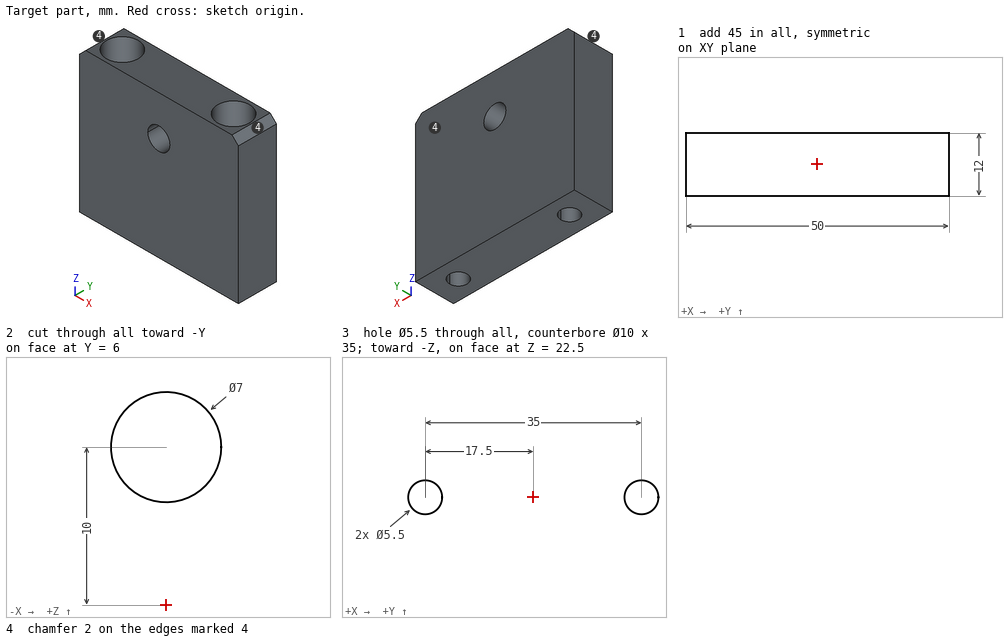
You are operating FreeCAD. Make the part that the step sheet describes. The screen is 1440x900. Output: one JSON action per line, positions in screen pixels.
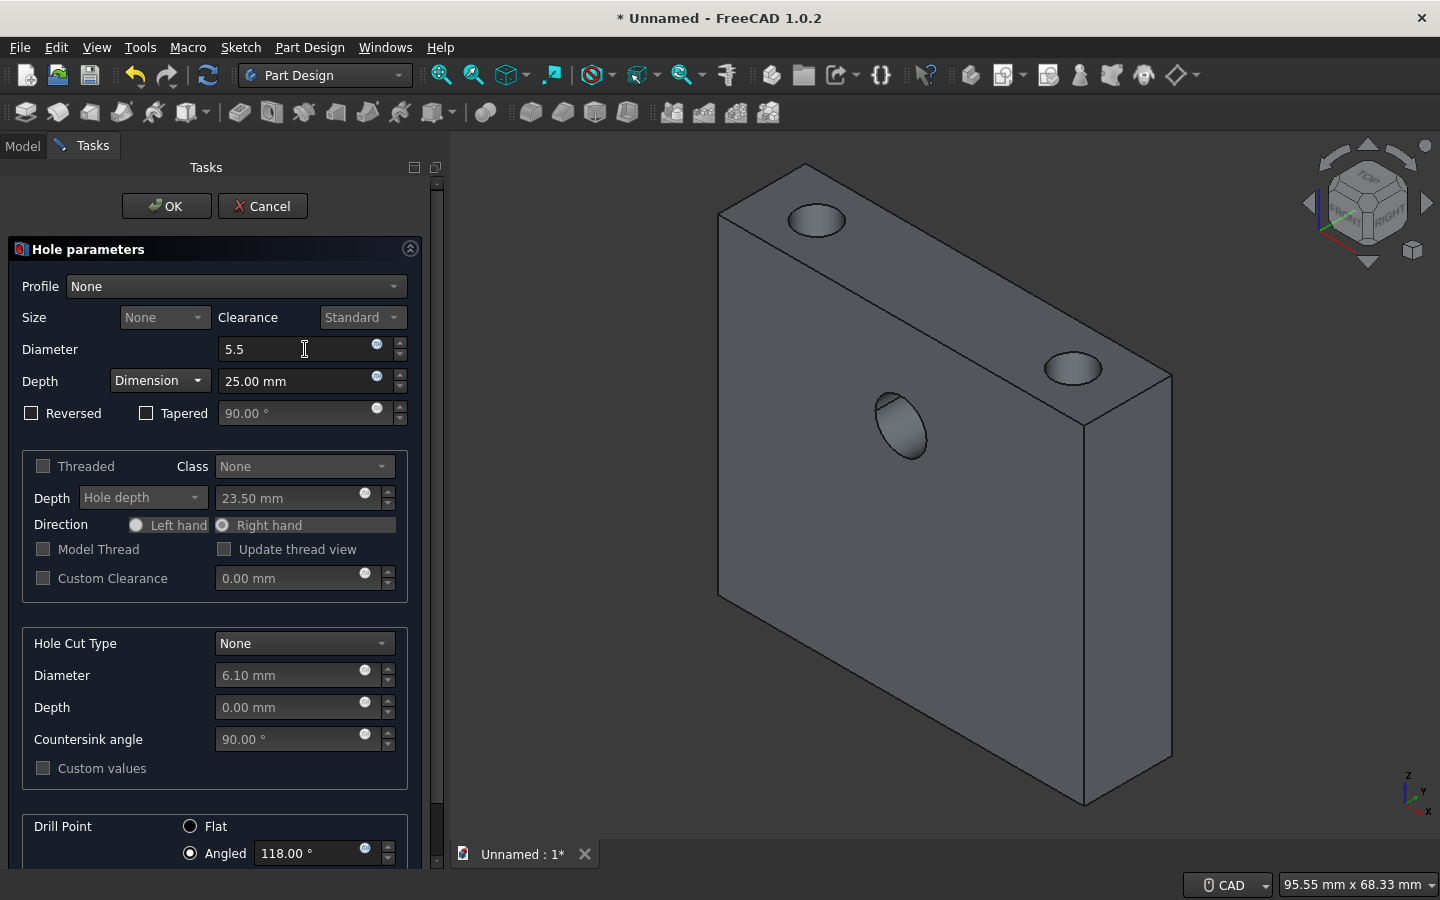
{"action": "left_click", "coordinate": [161, 380]}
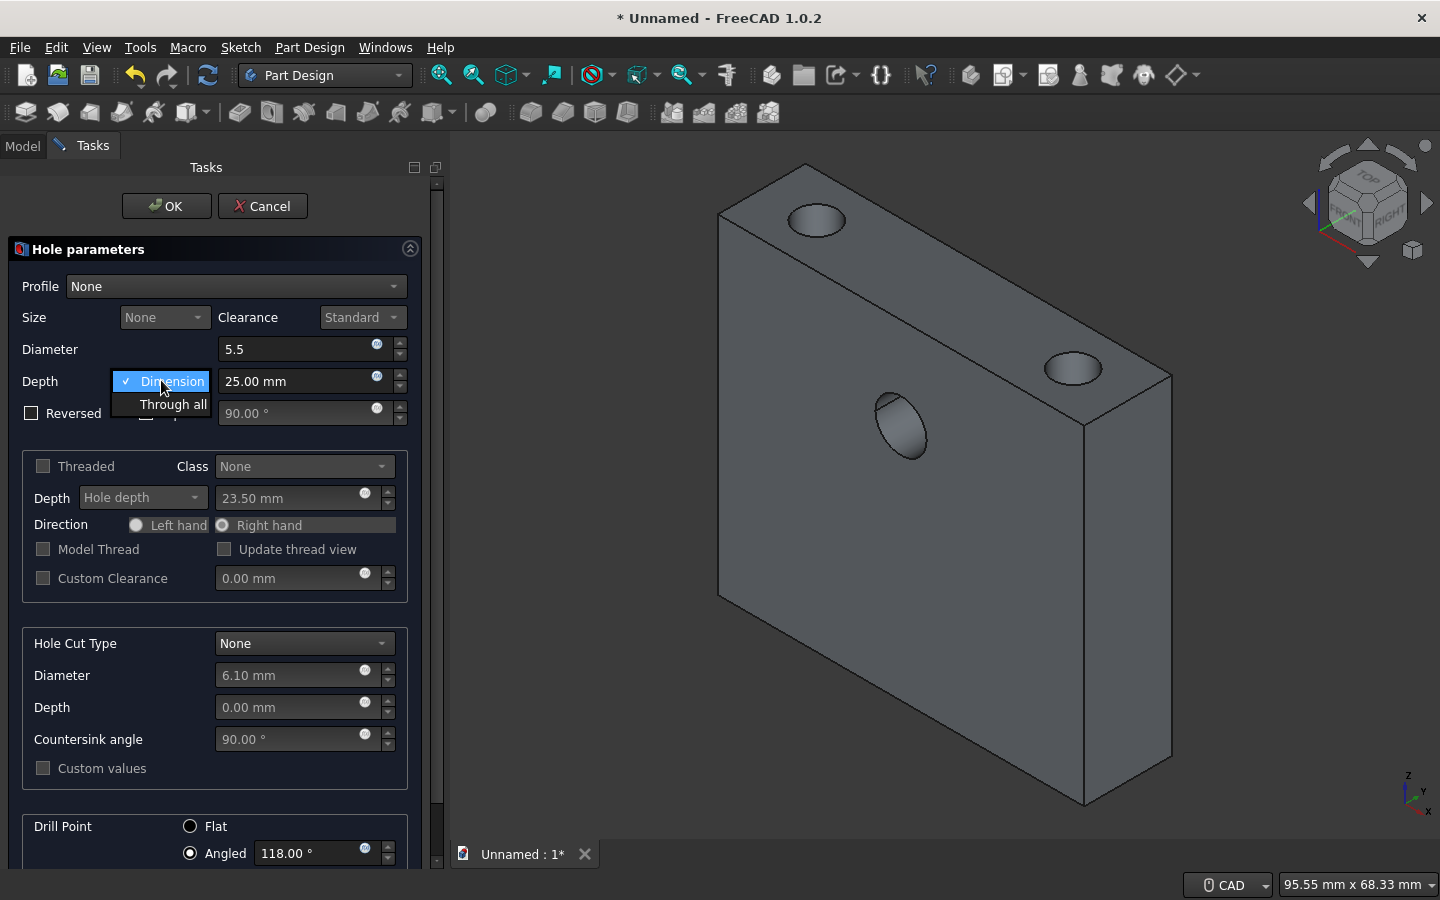
{"action": "left_click", "coordinate": [160, 404]}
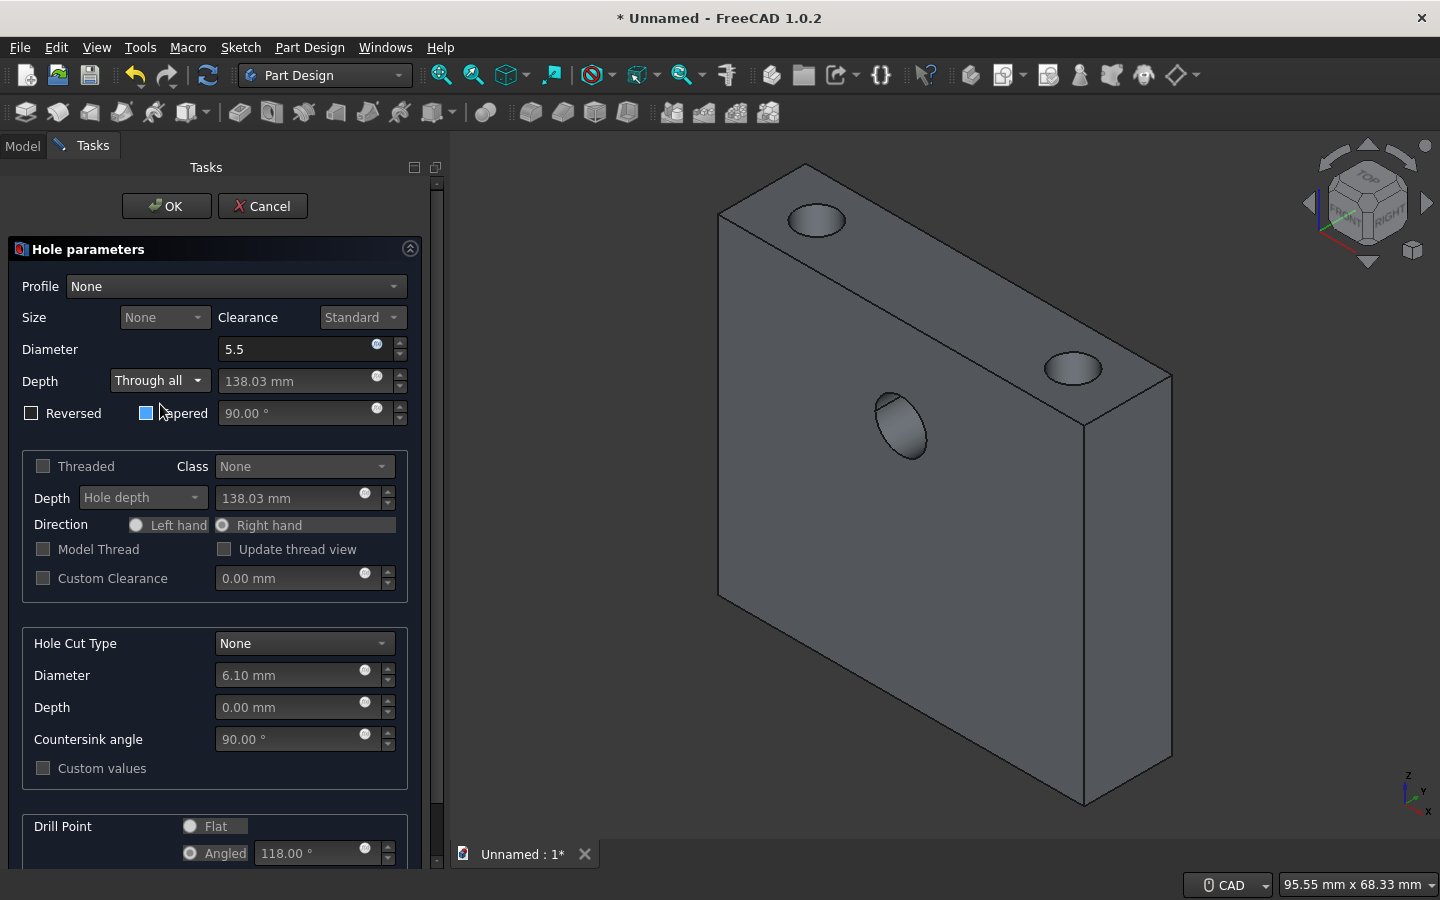
{"action": "left_click", "coordinate": [306, 644]}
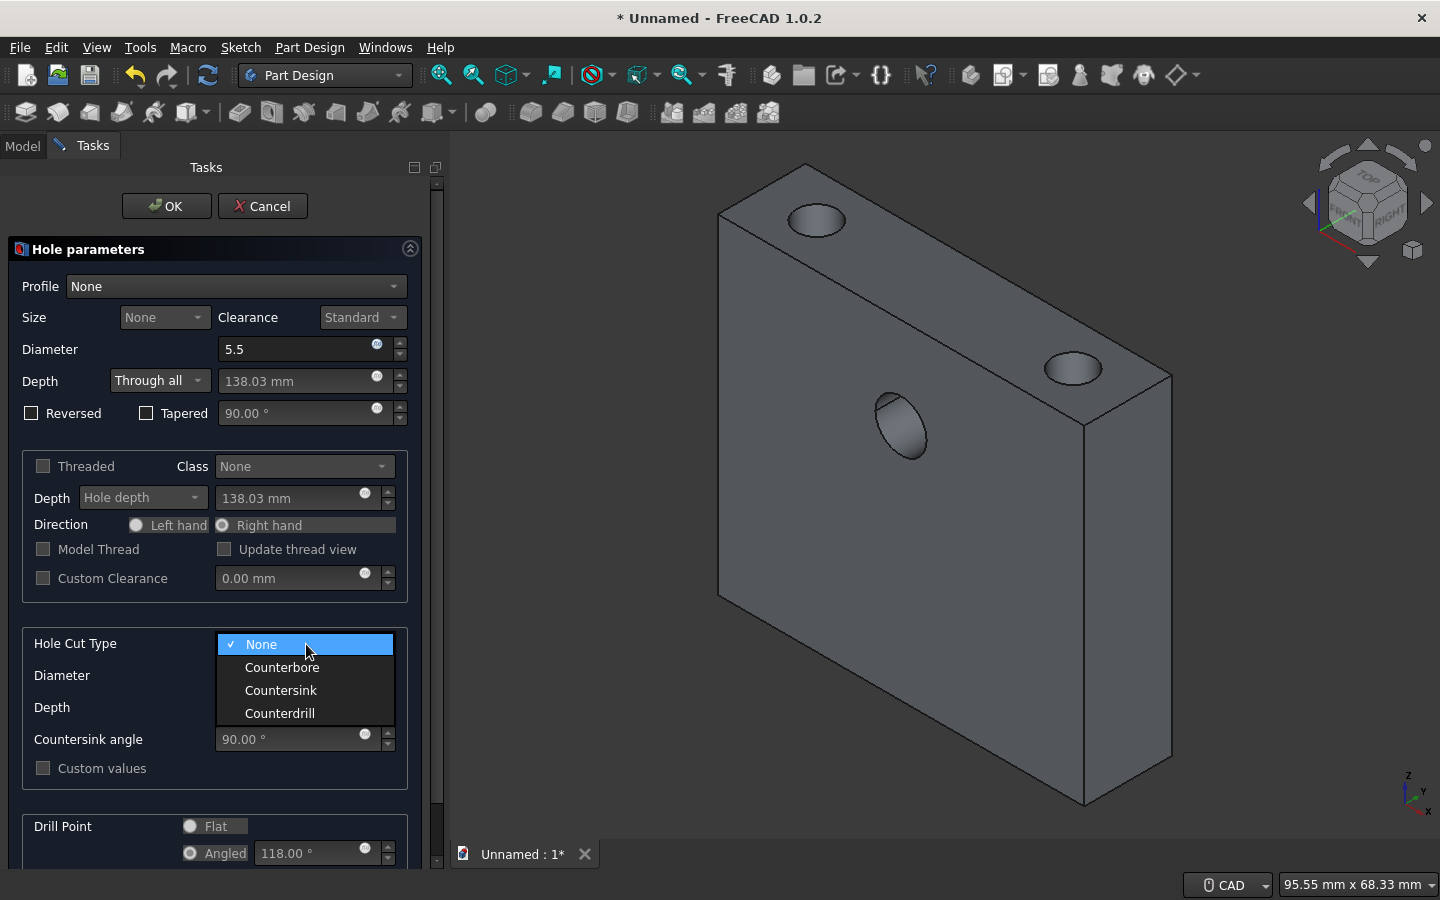
{"action": "left_click", "coordinate": [304, 668]}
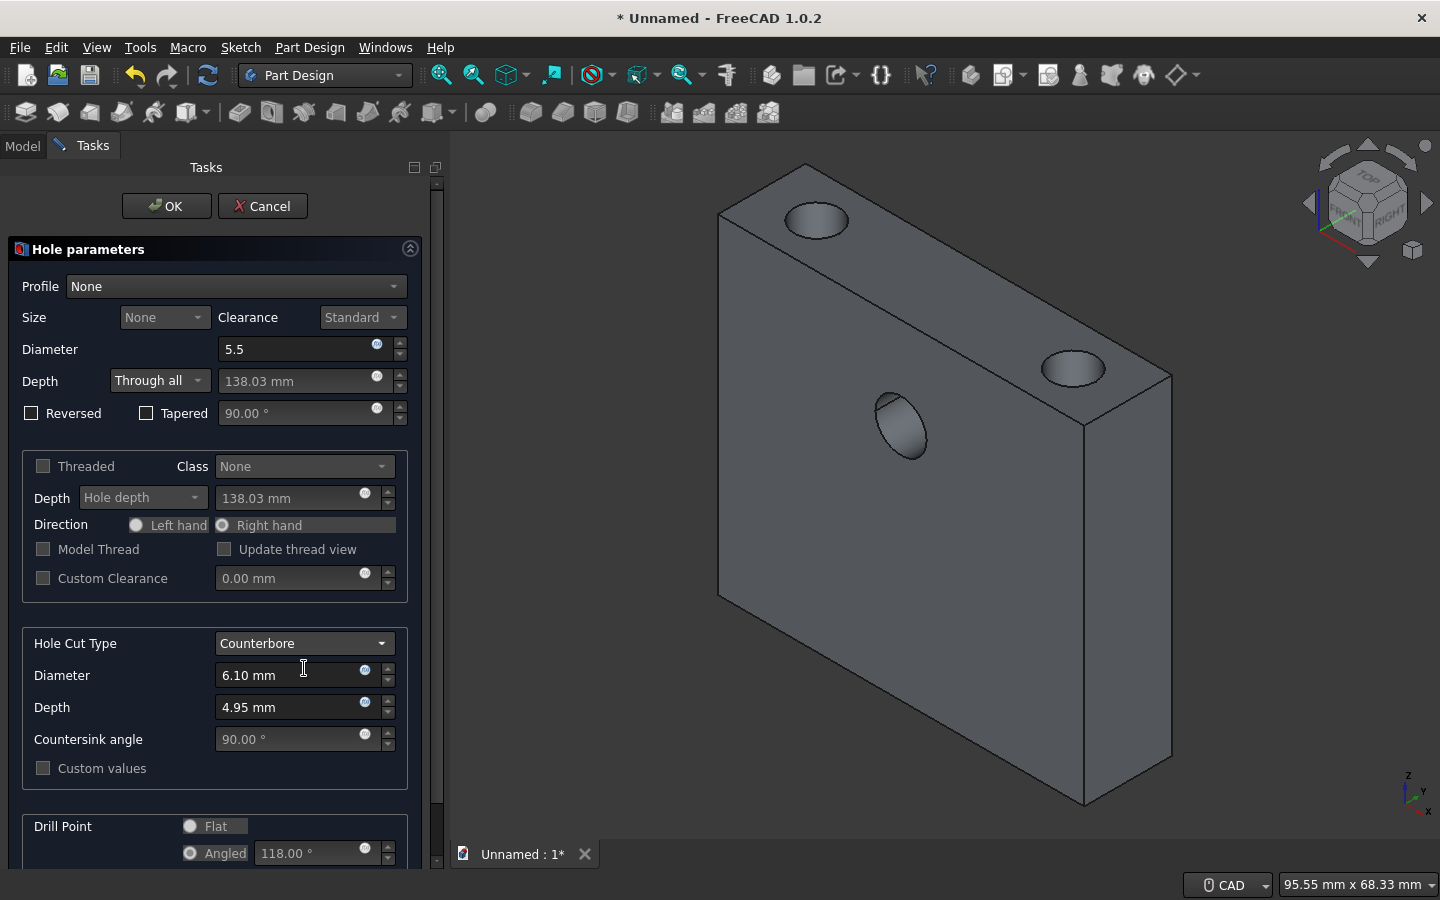
{"action": "triple_click", "coordinate": [298, 675]}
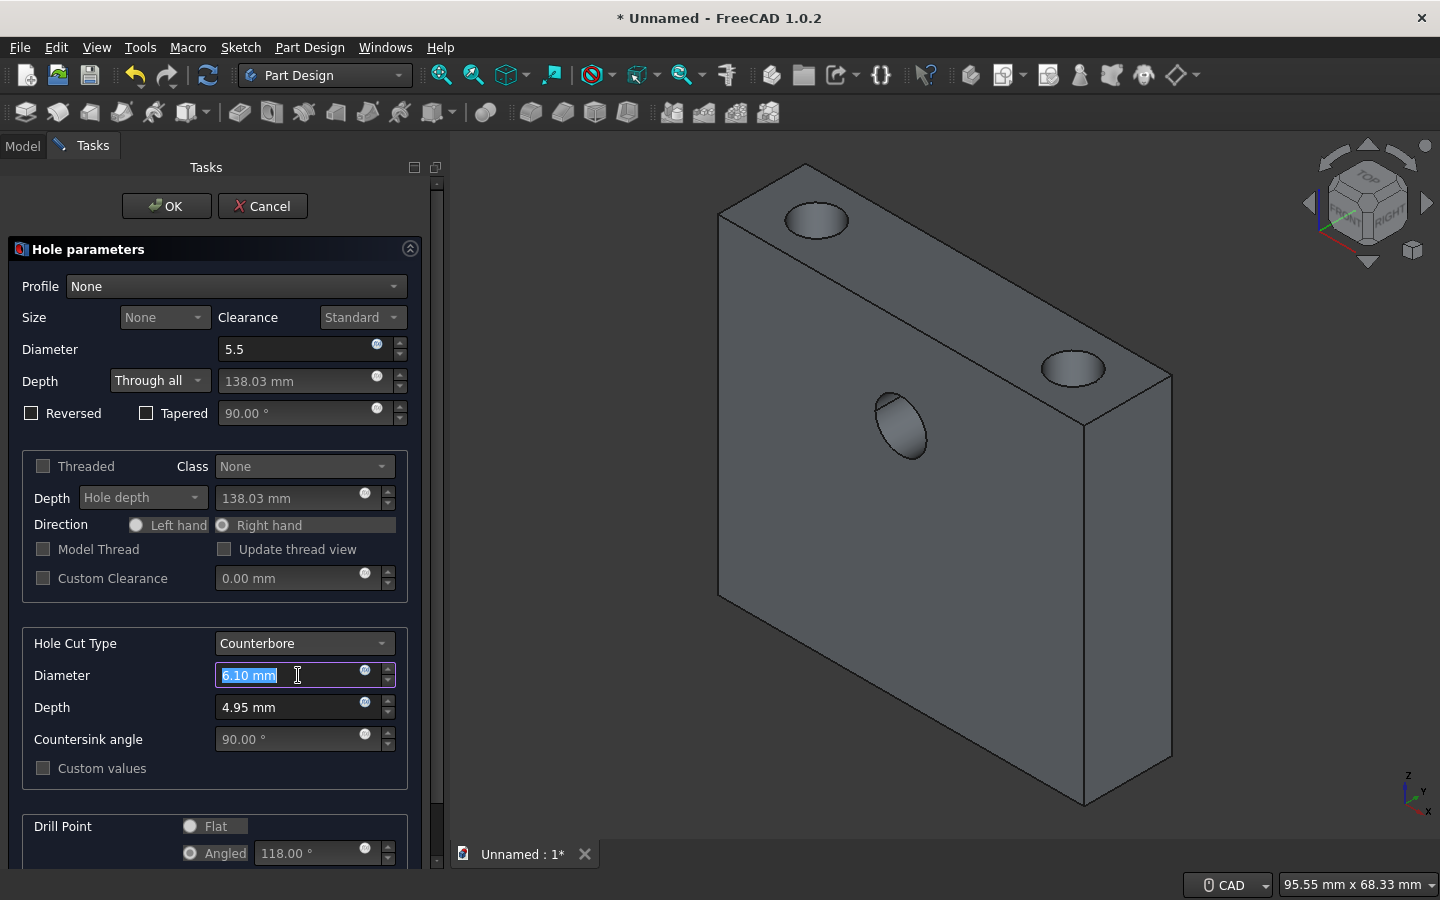
{"action": "type", "text": "10"}
{"action": "key", "text": "Tab"}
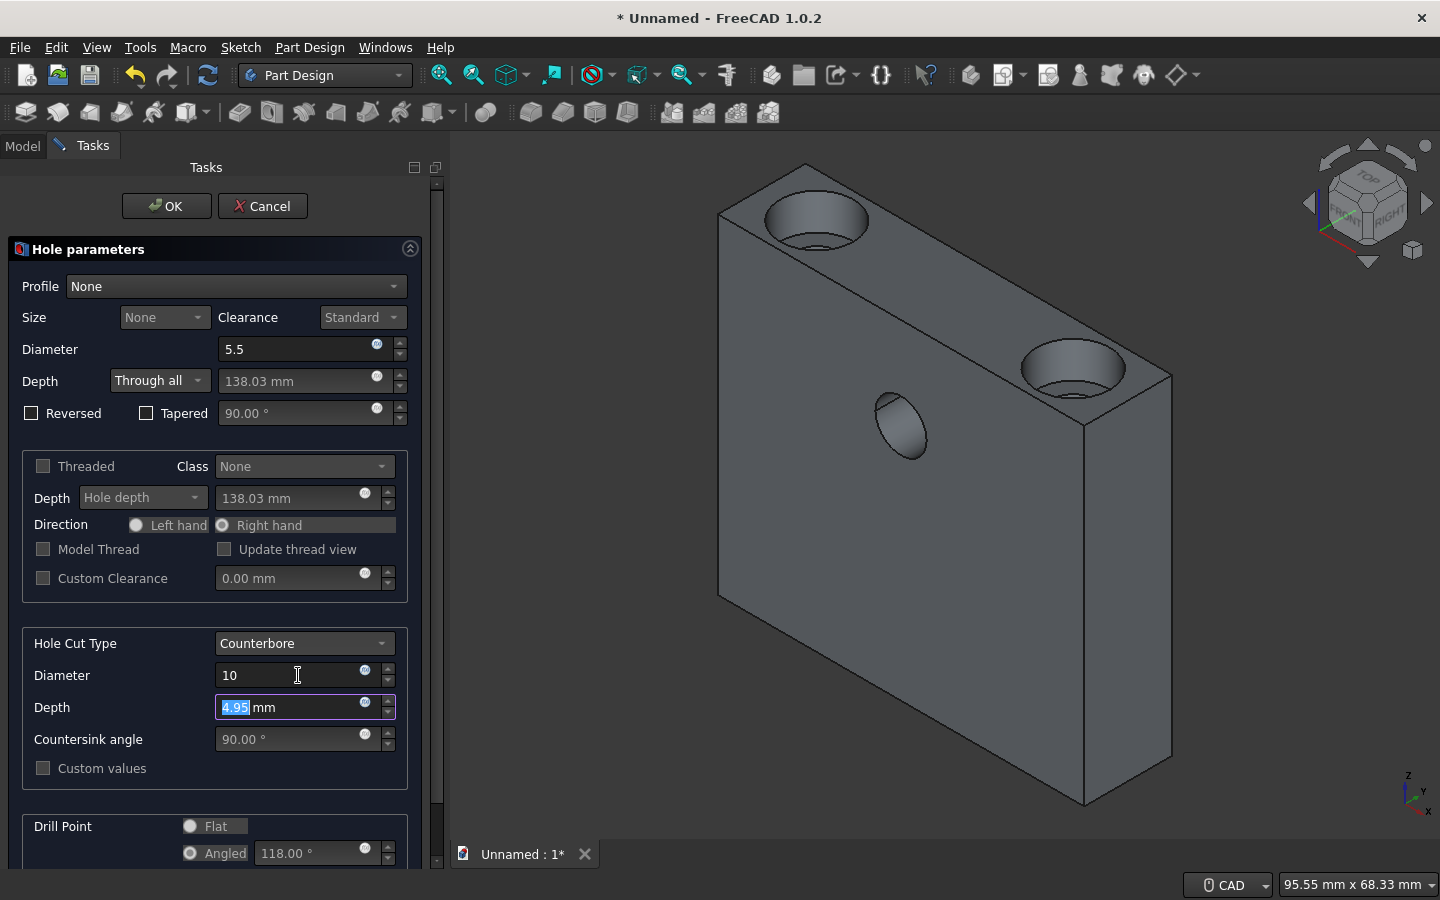
{"action": "type", "text": "35"}
{"action": "key", "text": "Tab"}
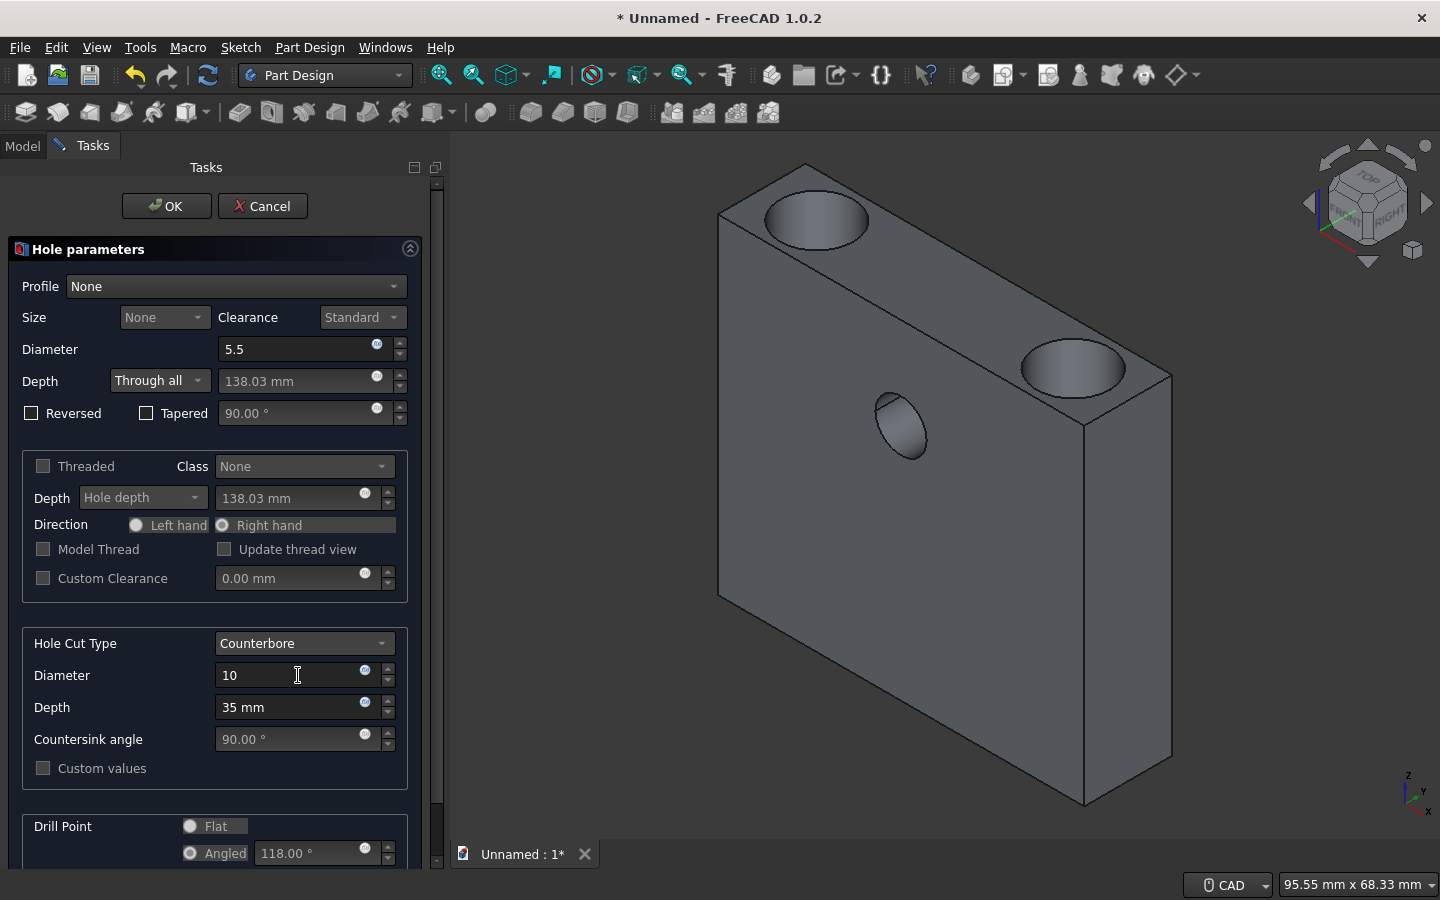
{"action": "left_click", "coordinate": [167, 206]}